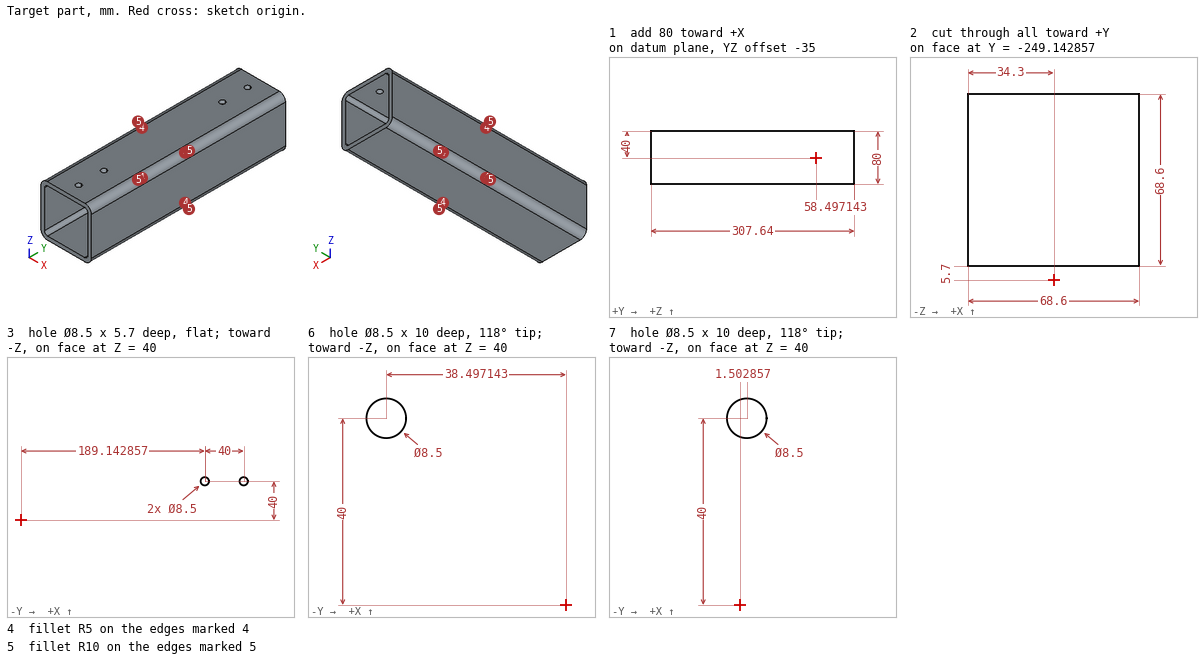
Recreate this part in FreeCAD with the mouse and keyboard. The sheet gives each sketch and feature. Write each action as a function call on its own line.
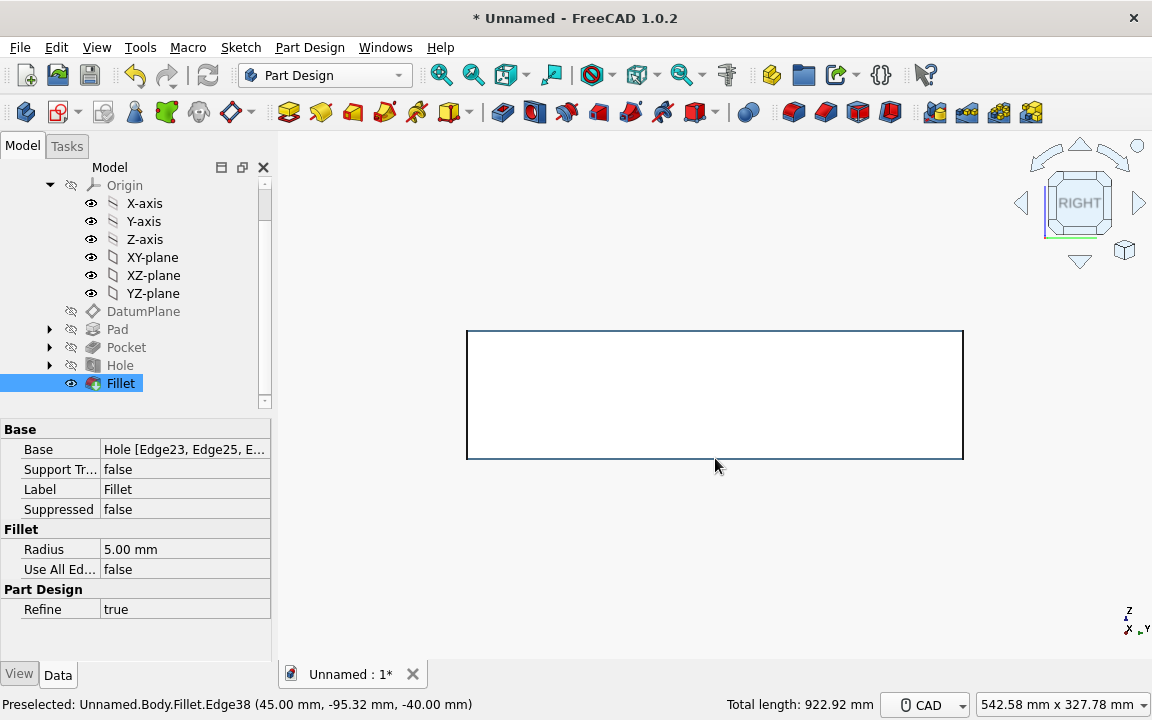
key(5)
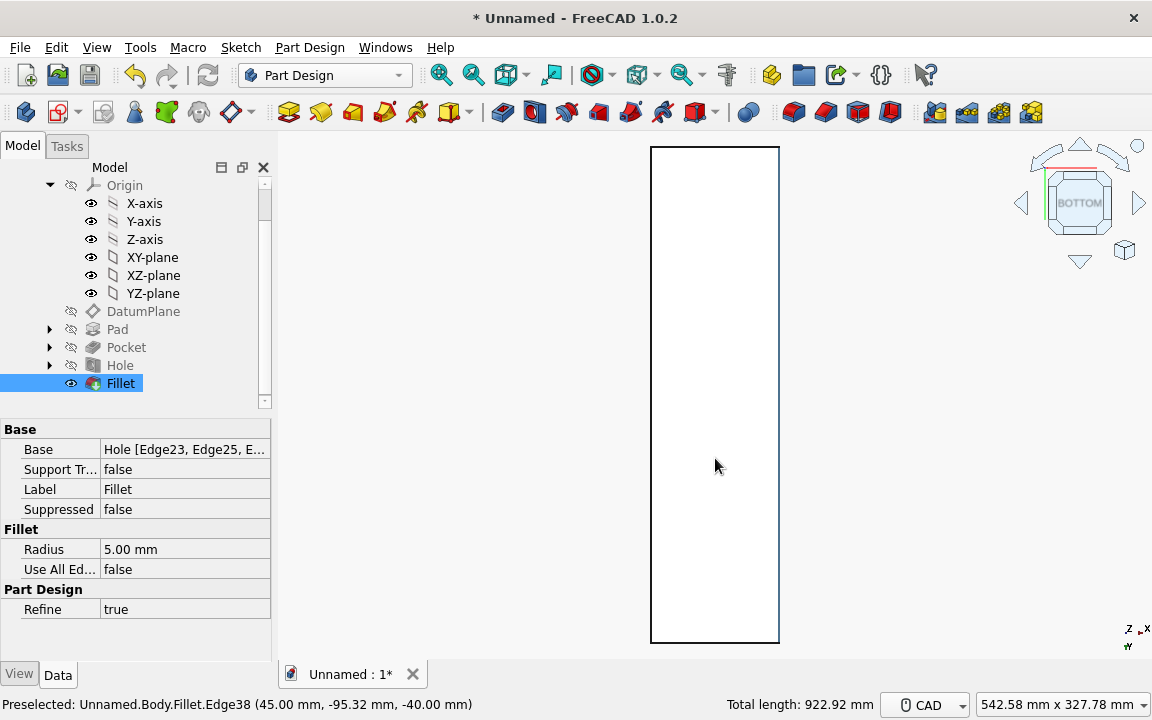
click(651, 394, ctrl)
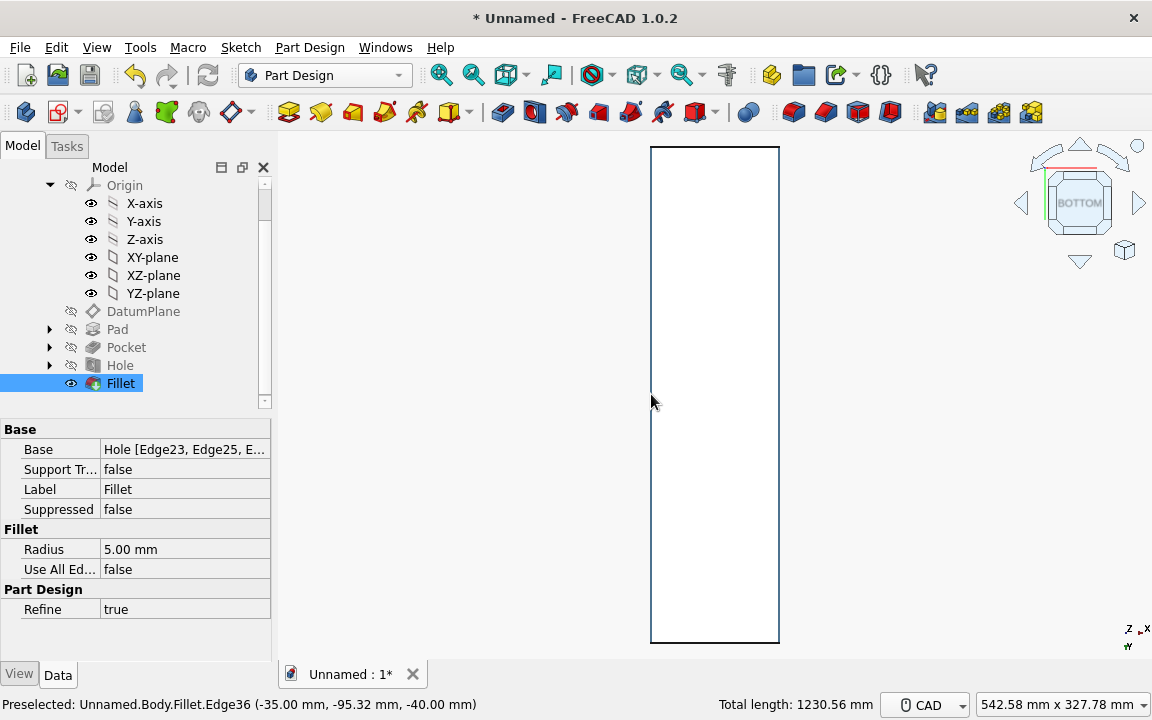
click(794, 112)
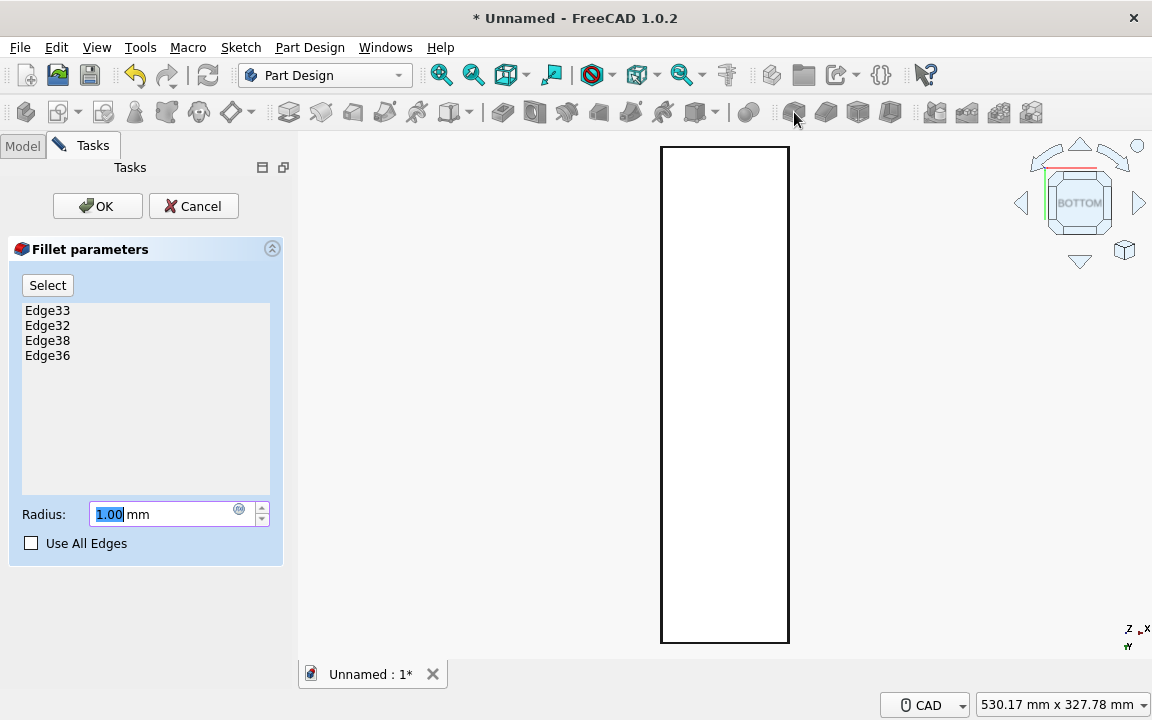
text(10)
key(Tab)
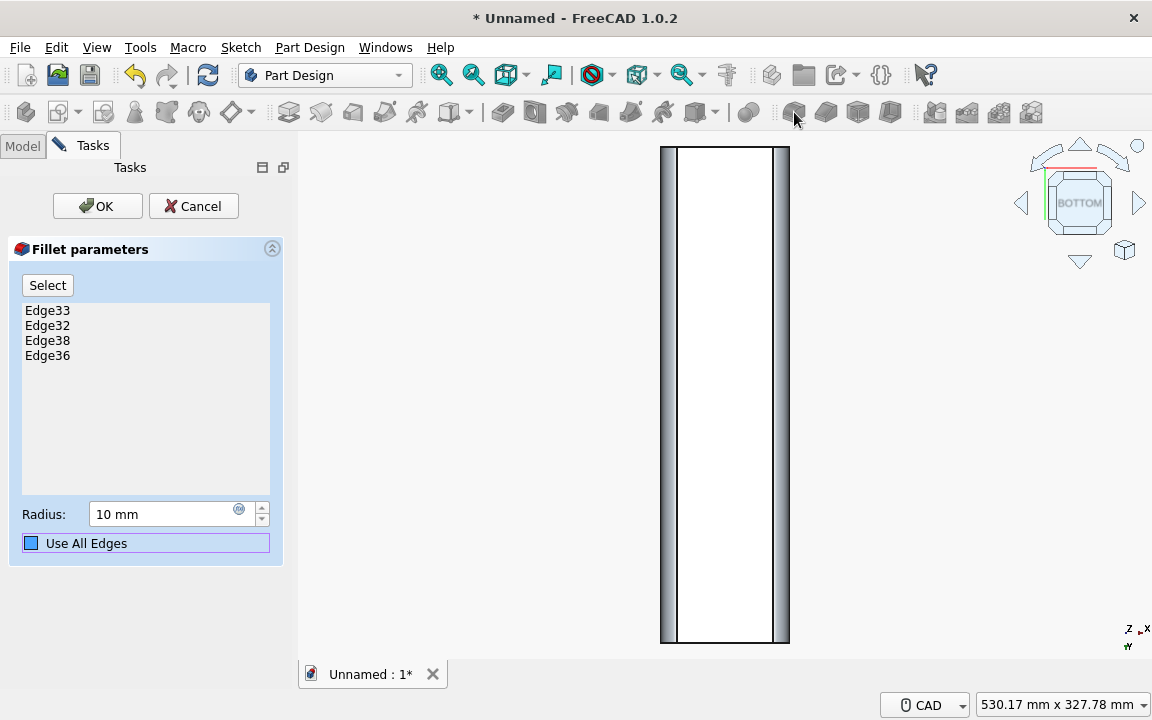
click(98, 206)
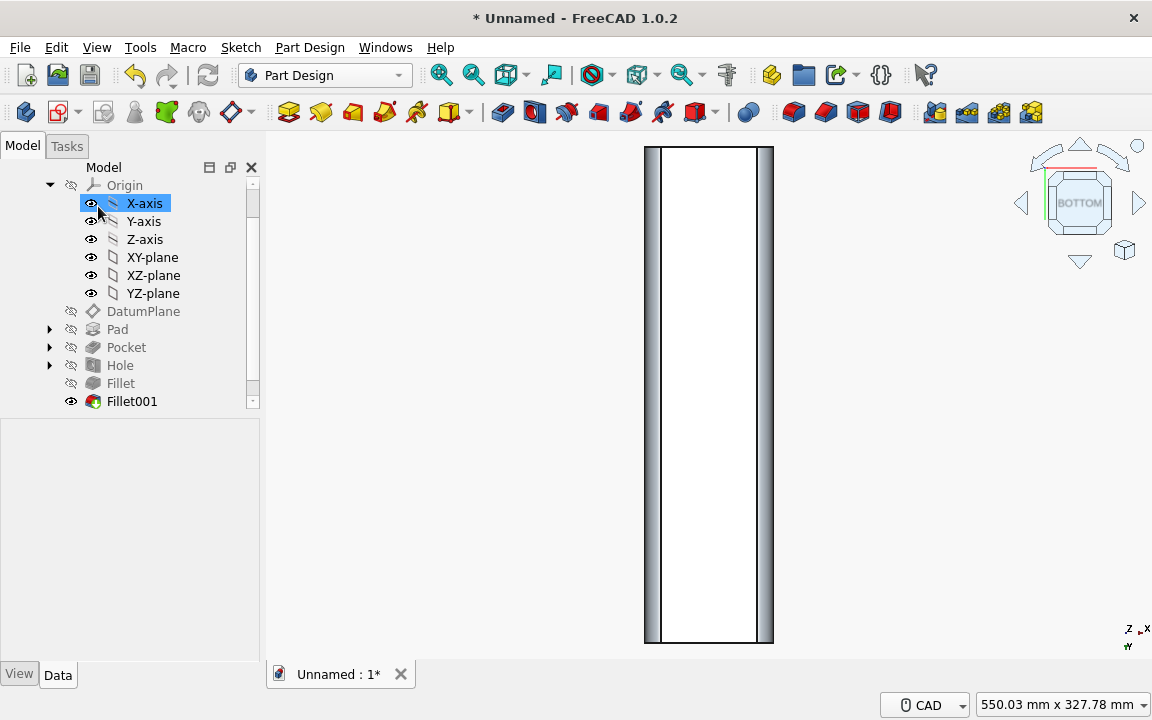
key(0)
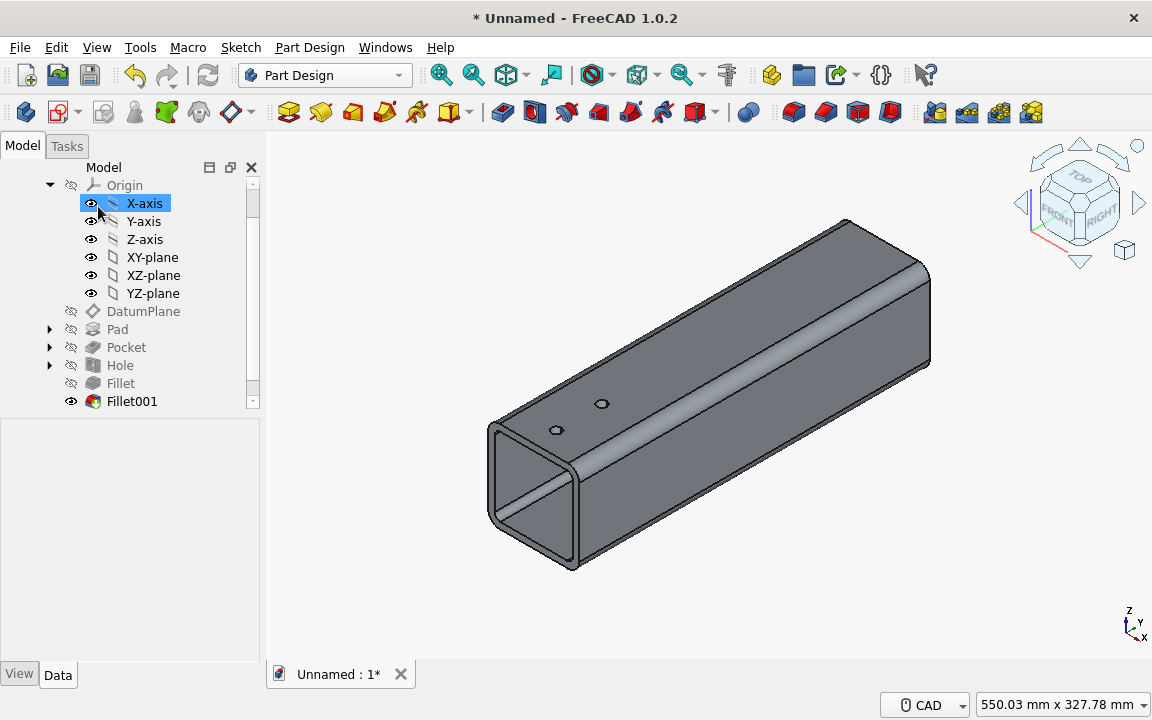
click(659, 370)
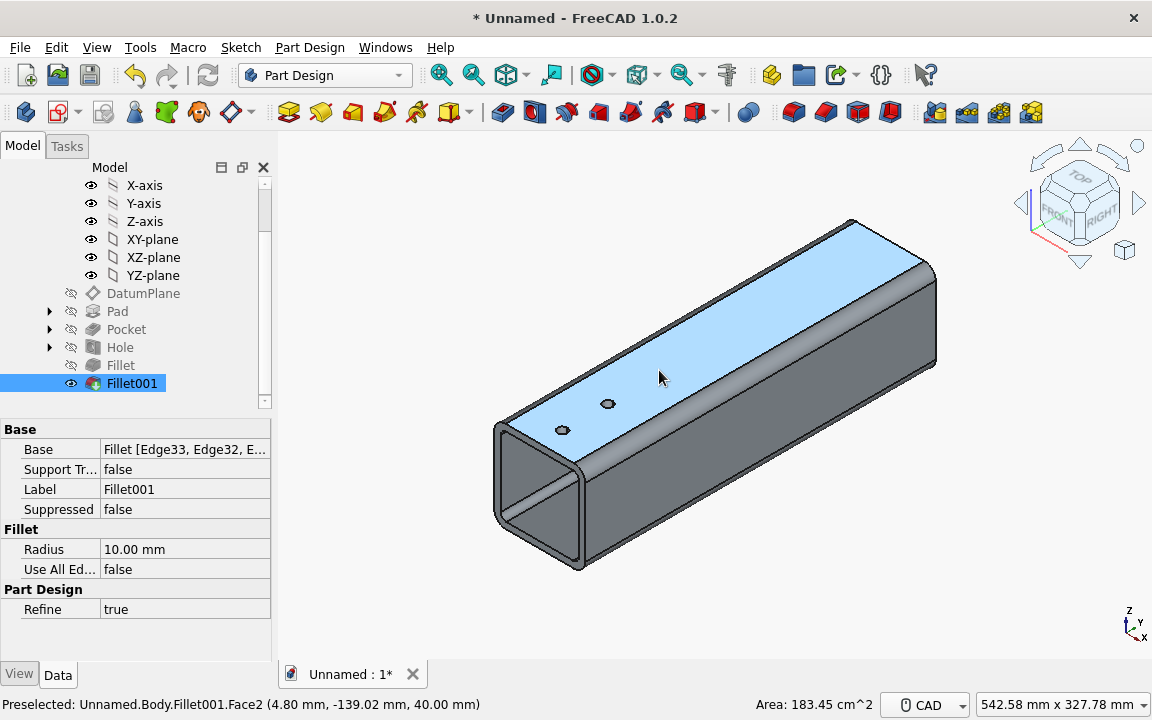
click(58, 112)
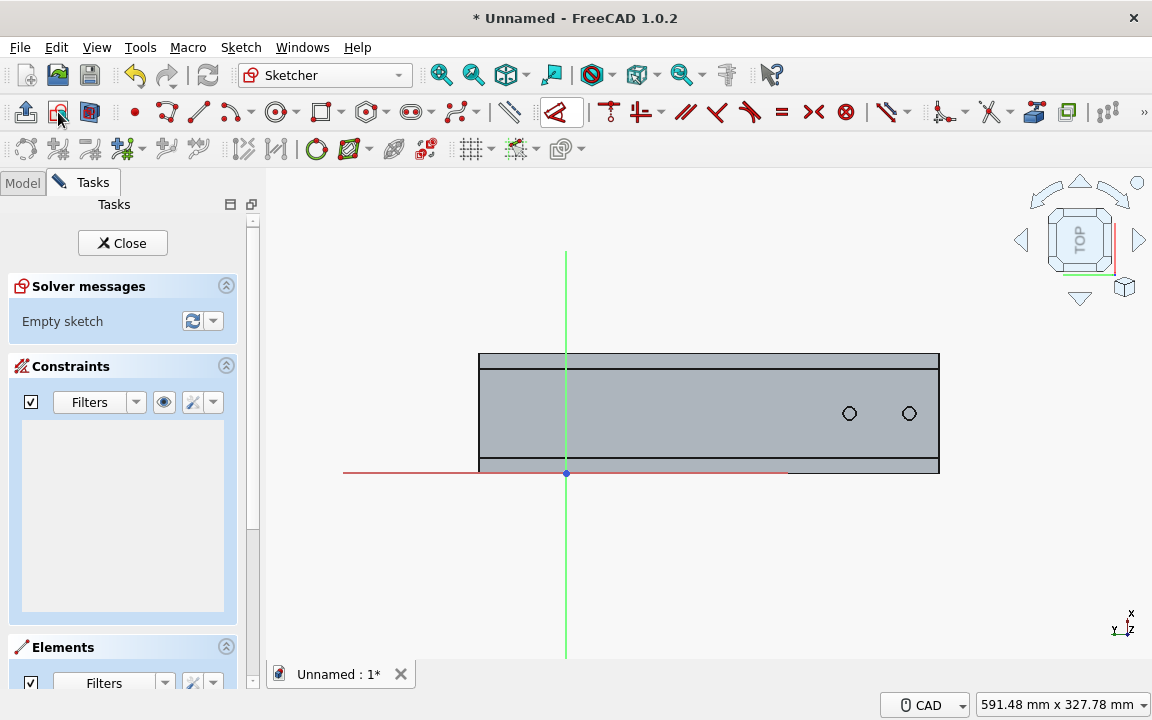
scroll(502, 414, up, 15)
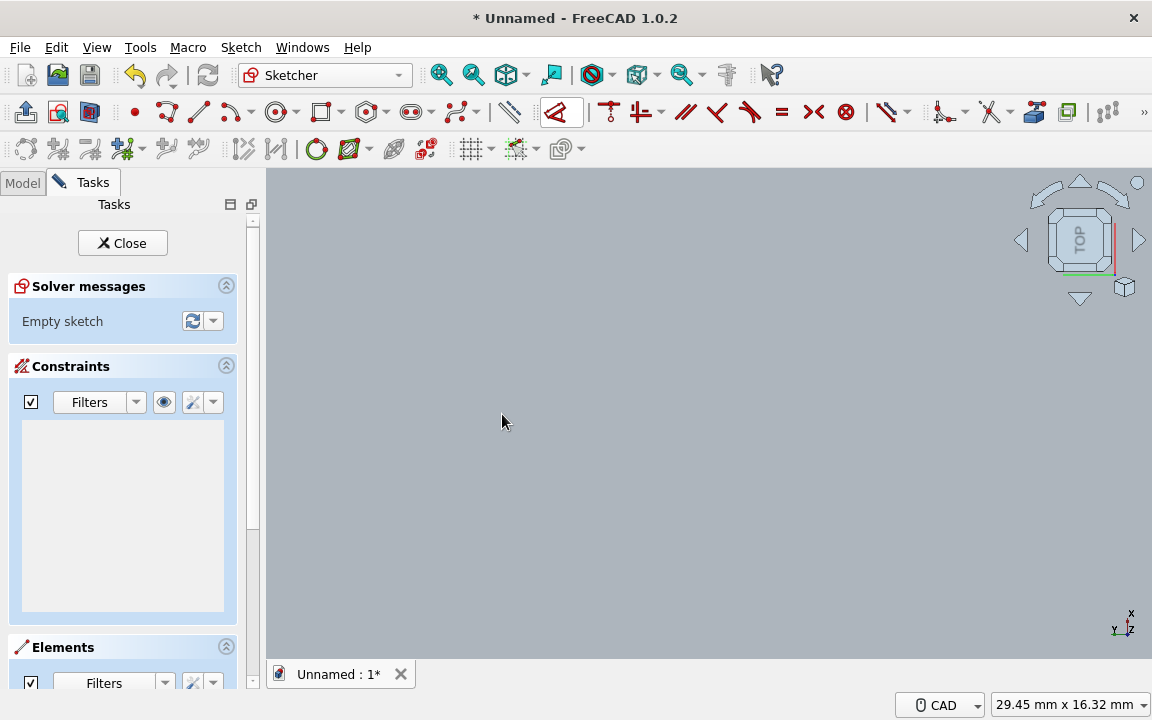
key(g)
key(c)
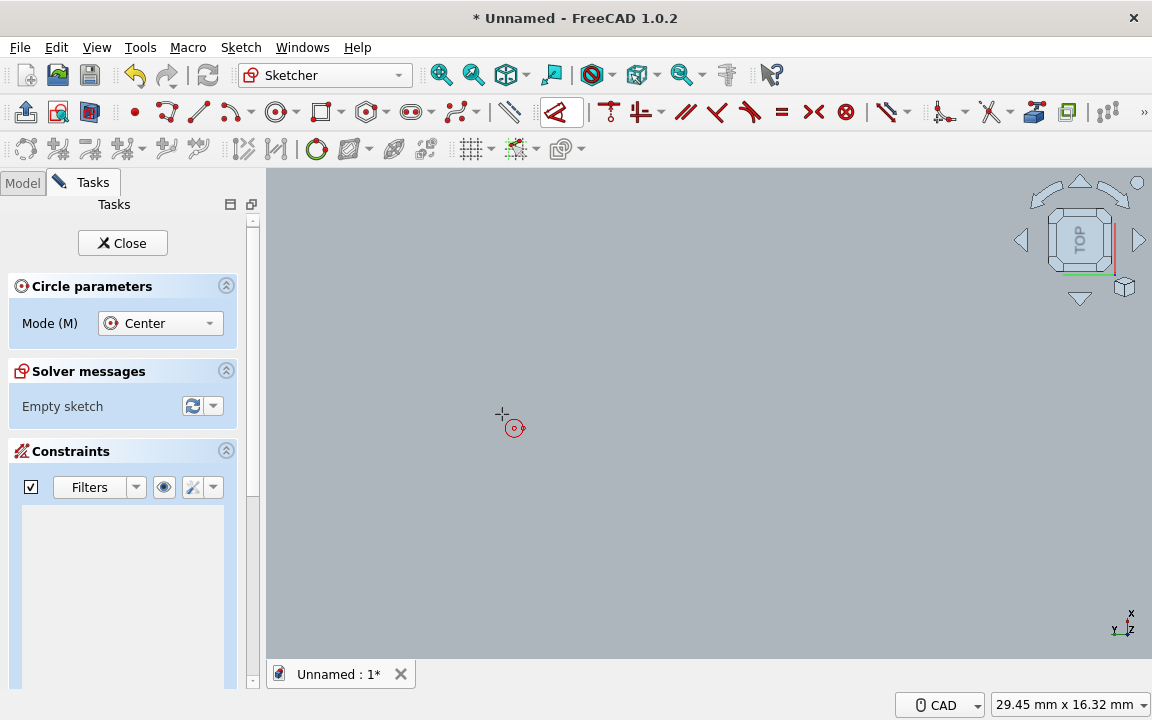
click(628, 394)
move(719, 304)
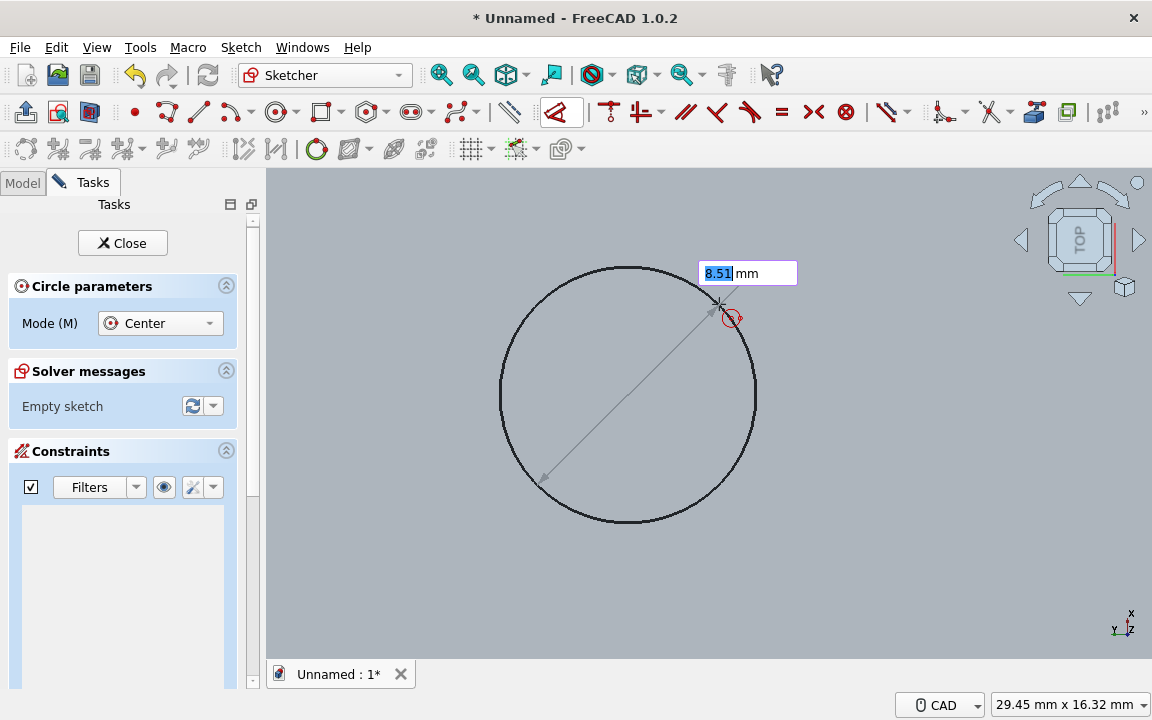
text(8.5)
key(Return)
key(Escape)